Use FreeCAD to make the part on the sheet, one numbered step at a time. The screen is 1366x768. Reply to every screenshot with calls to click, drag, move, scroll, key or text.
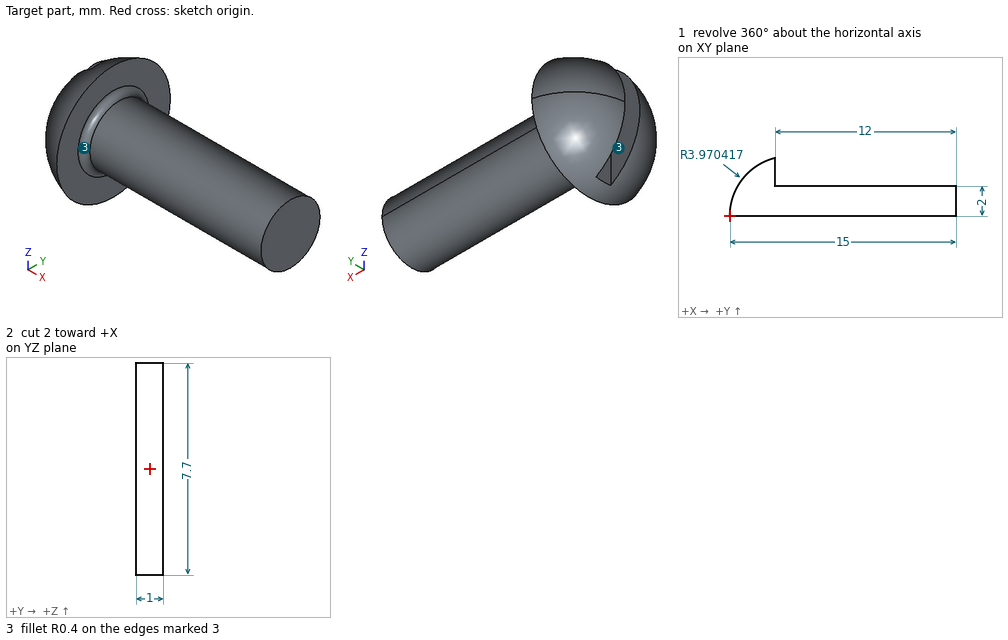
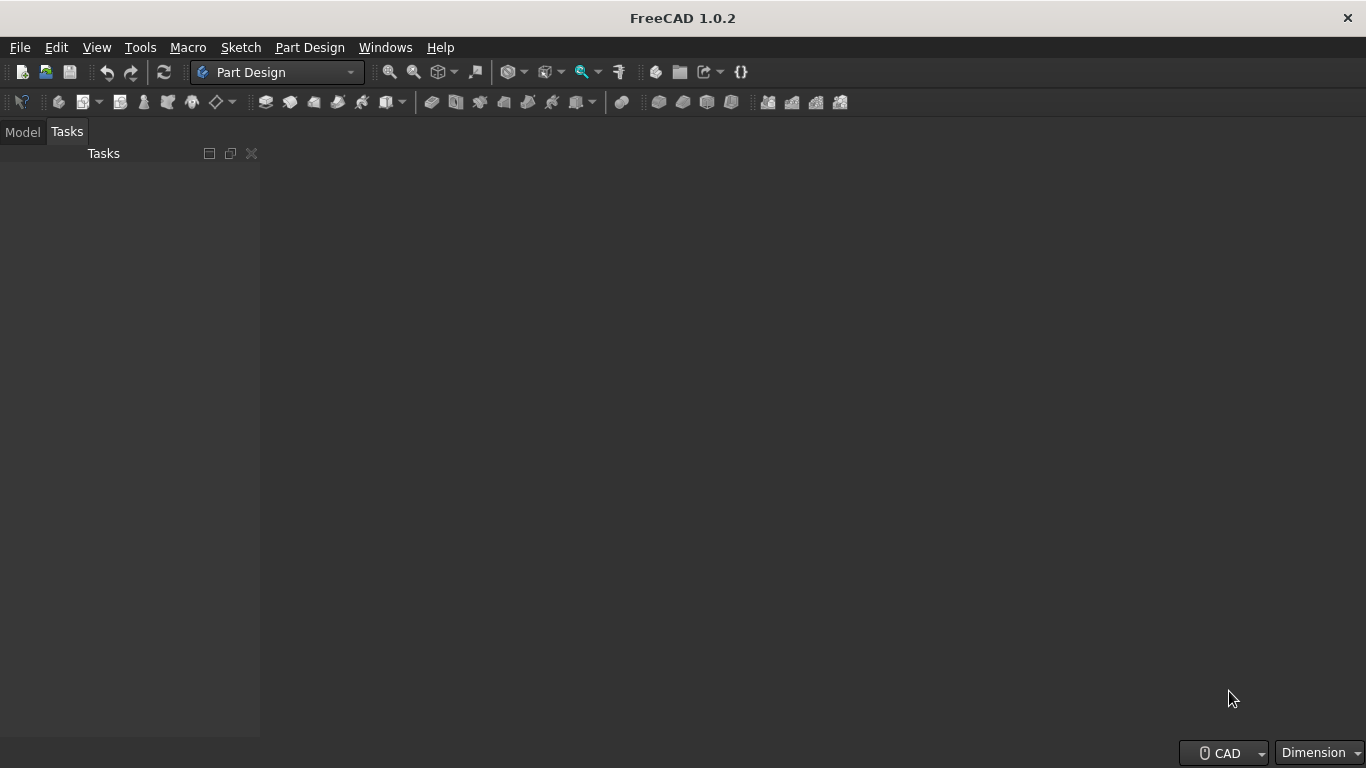
click(22, 72)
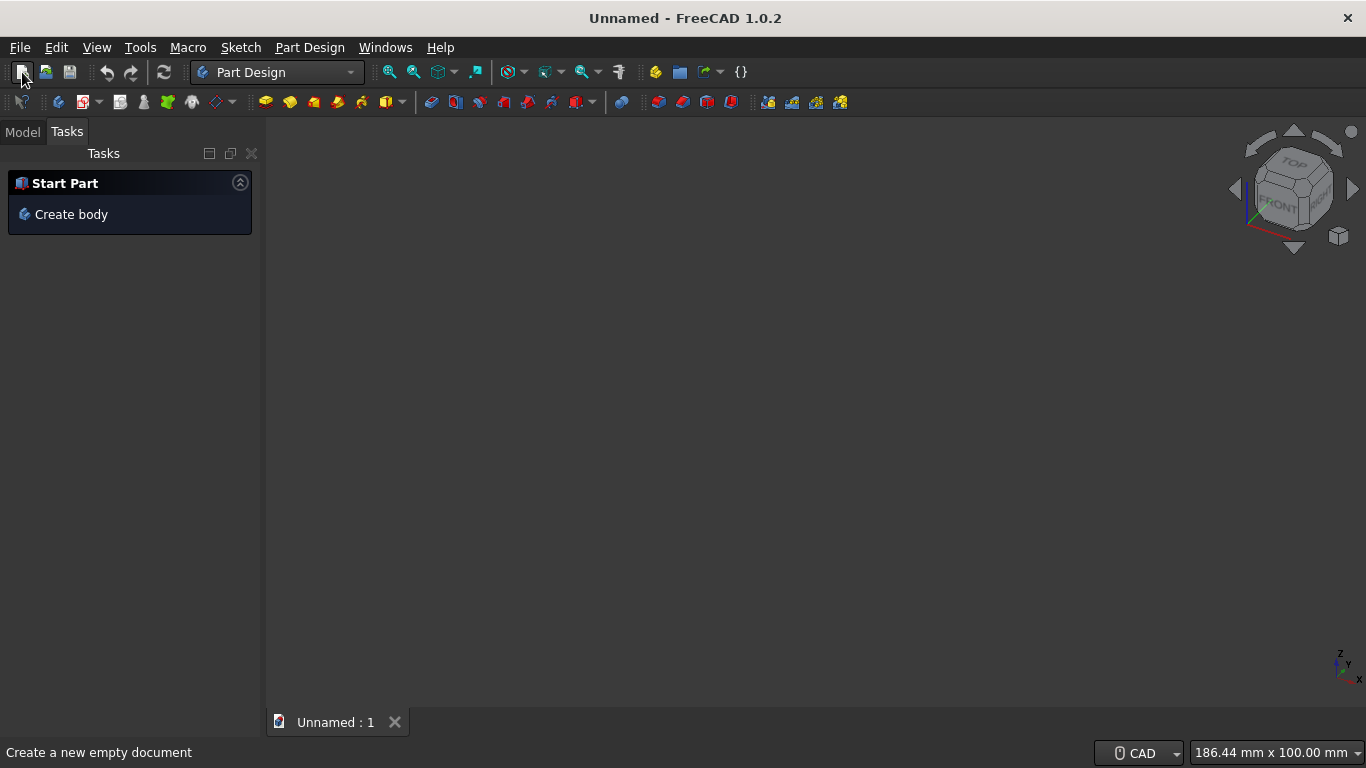
click(84, 102)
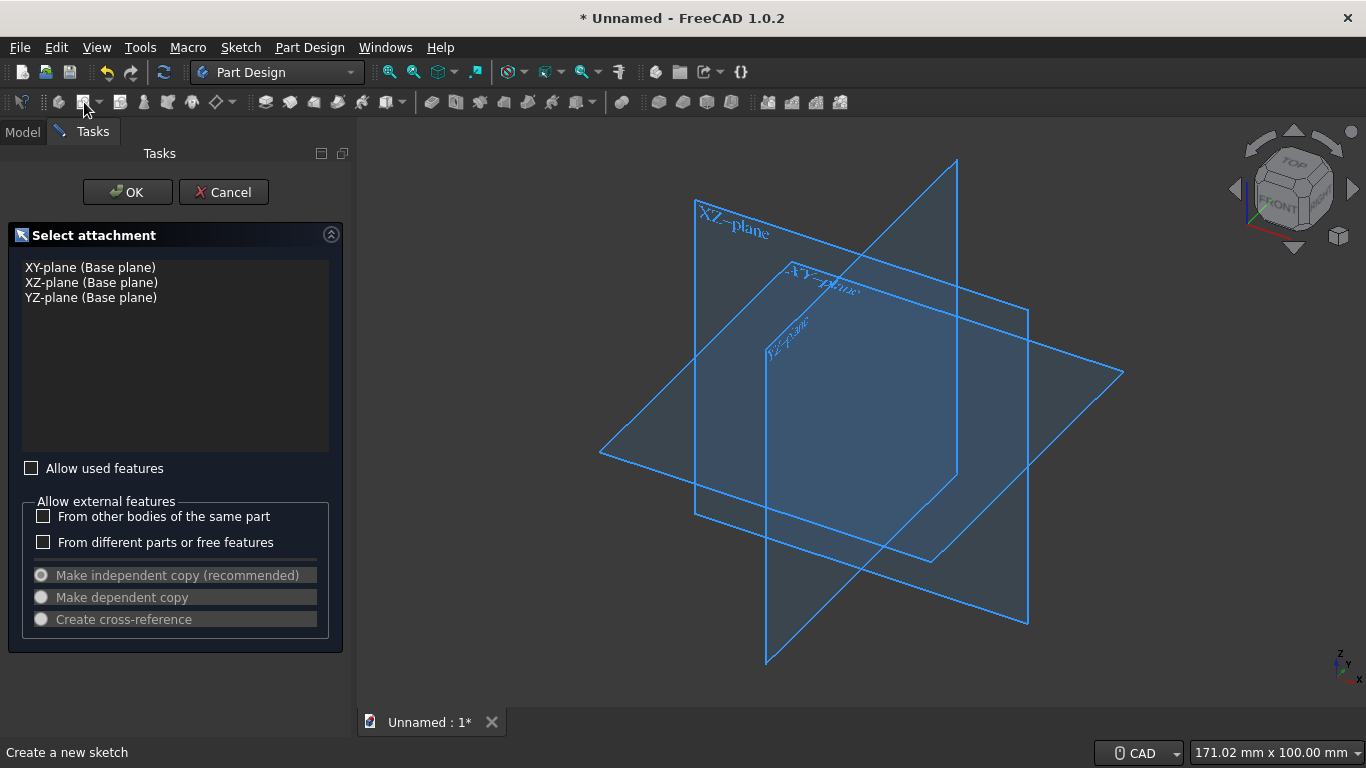
click(82, 268)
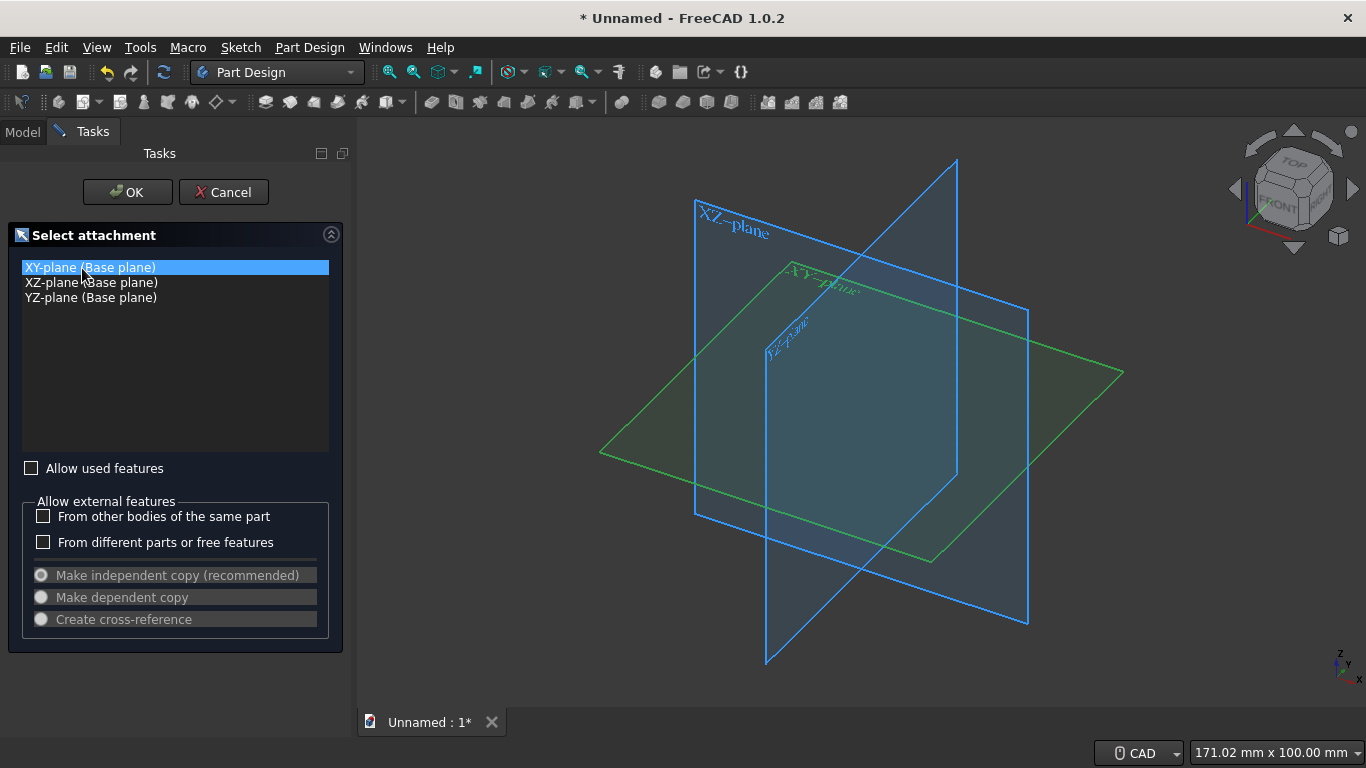
click(128, 192)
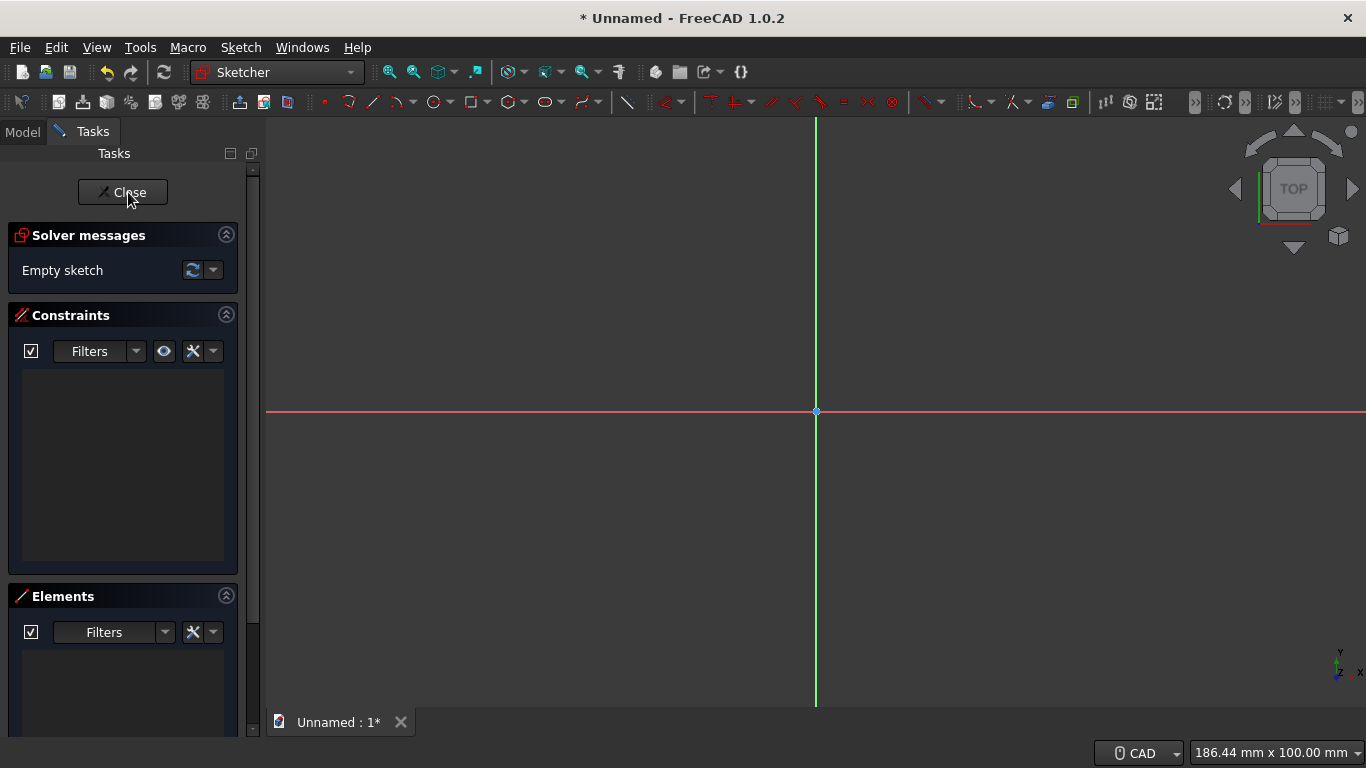
scroll(878, 399, up, 10)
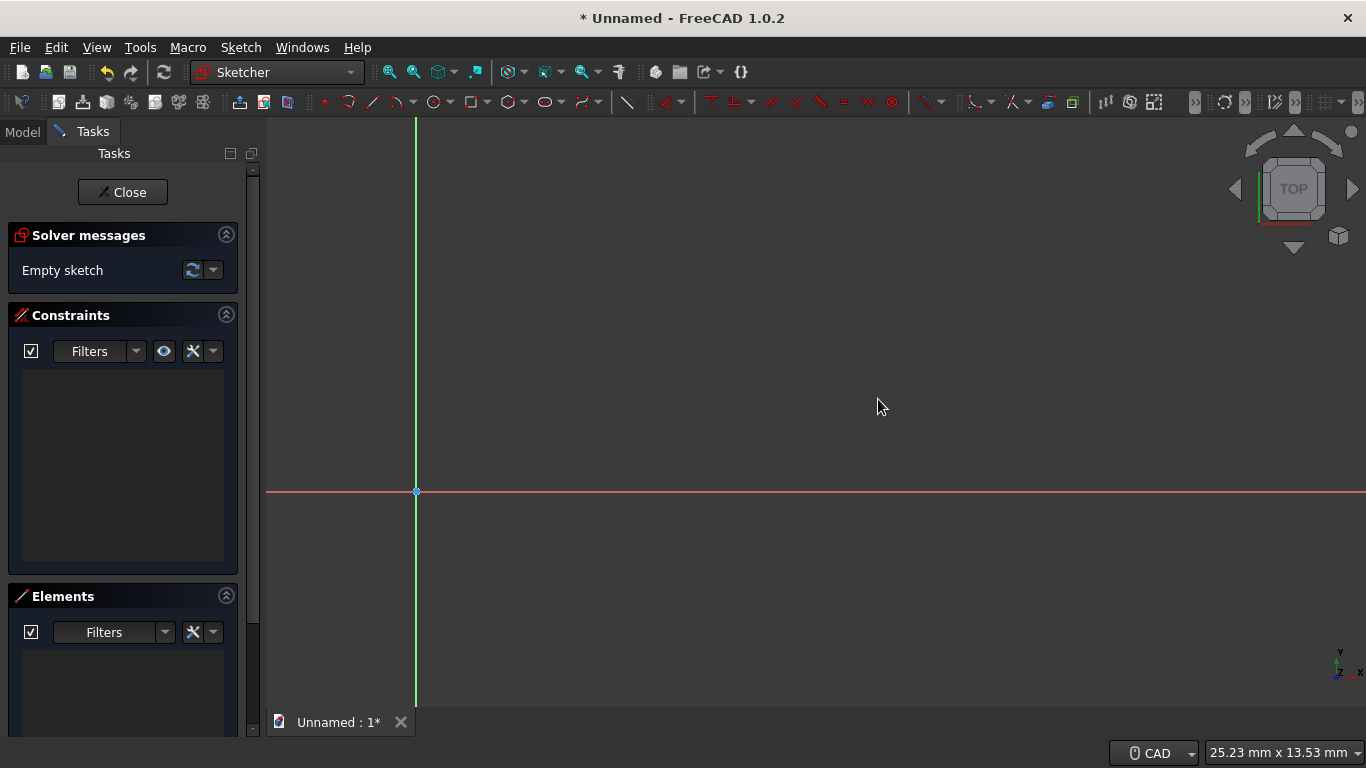
click(350, 102)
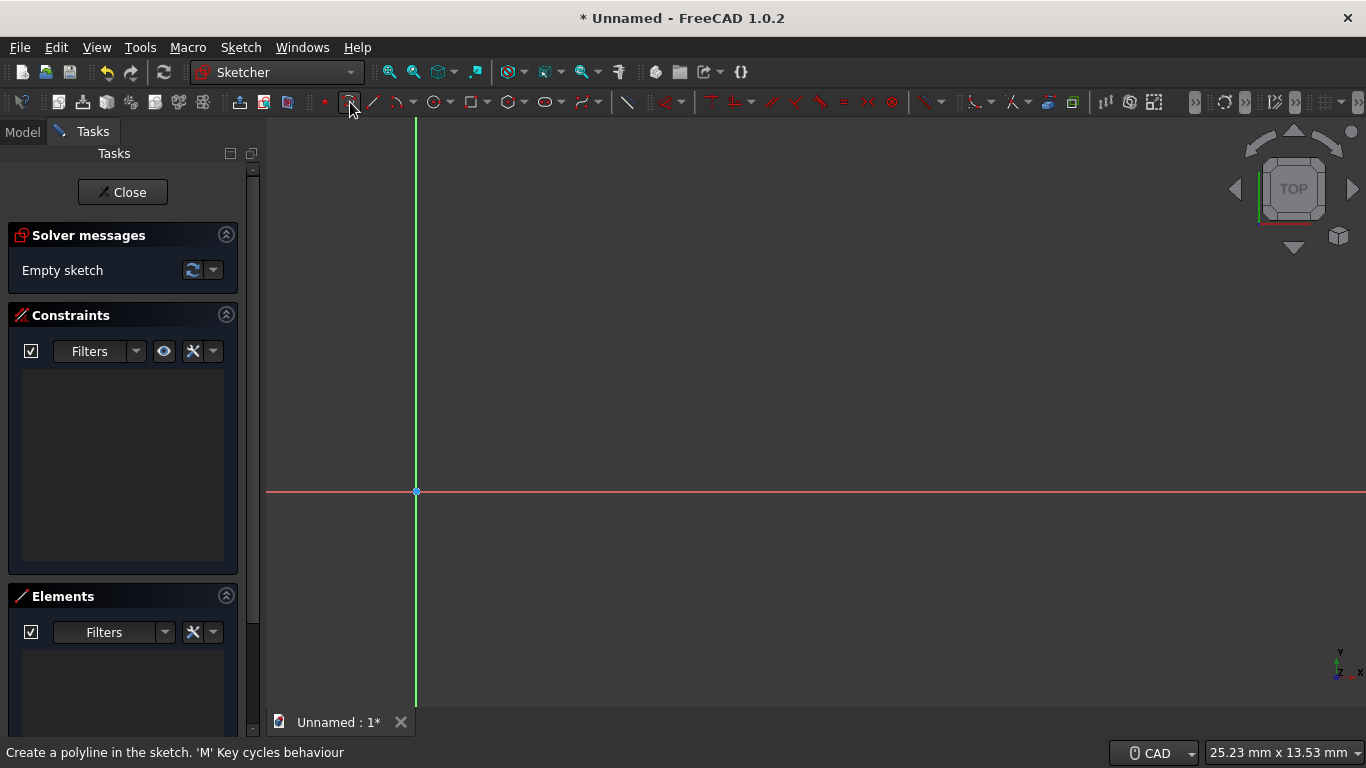
click(416, 492)
click(1070, 483)
click(1070, 405)
click(547, 405)
click(547, 324)
right_click(547, 324)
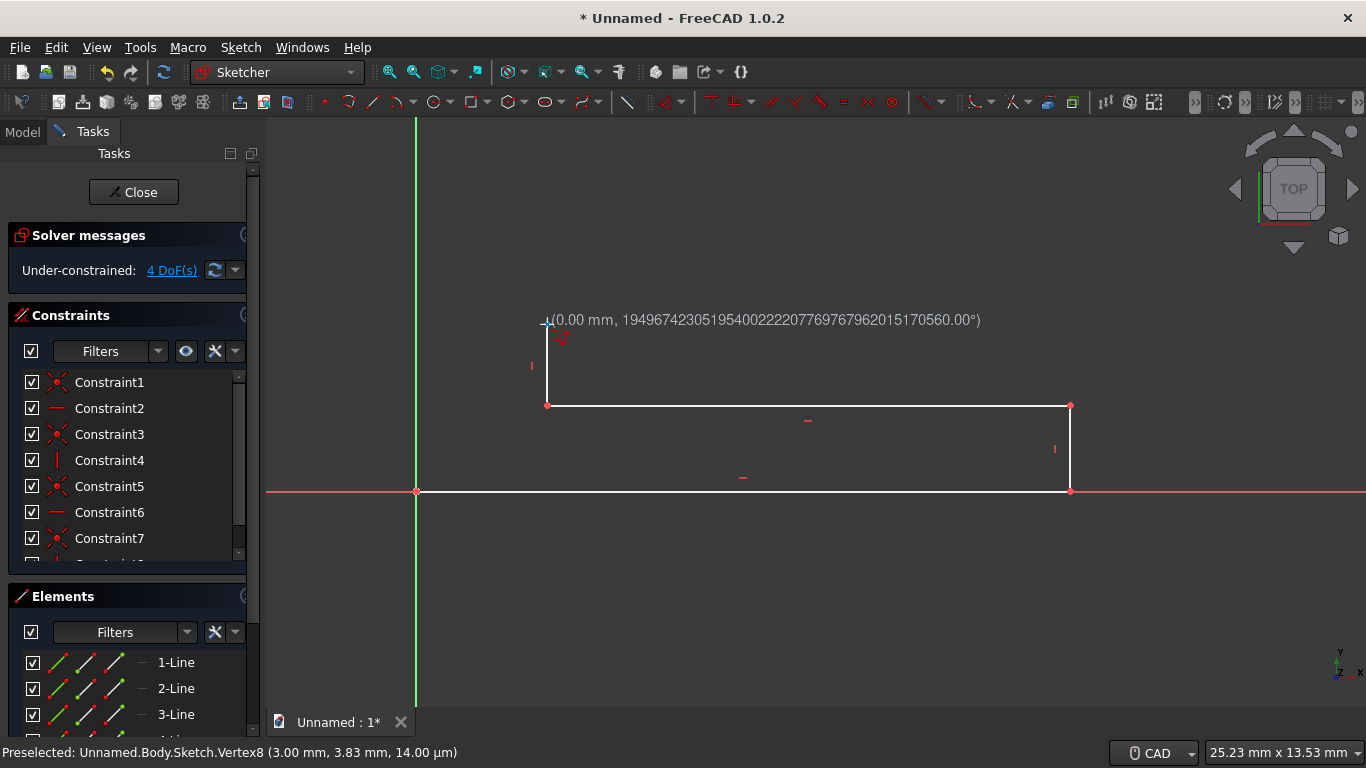
key(g)
key(3)
key(a)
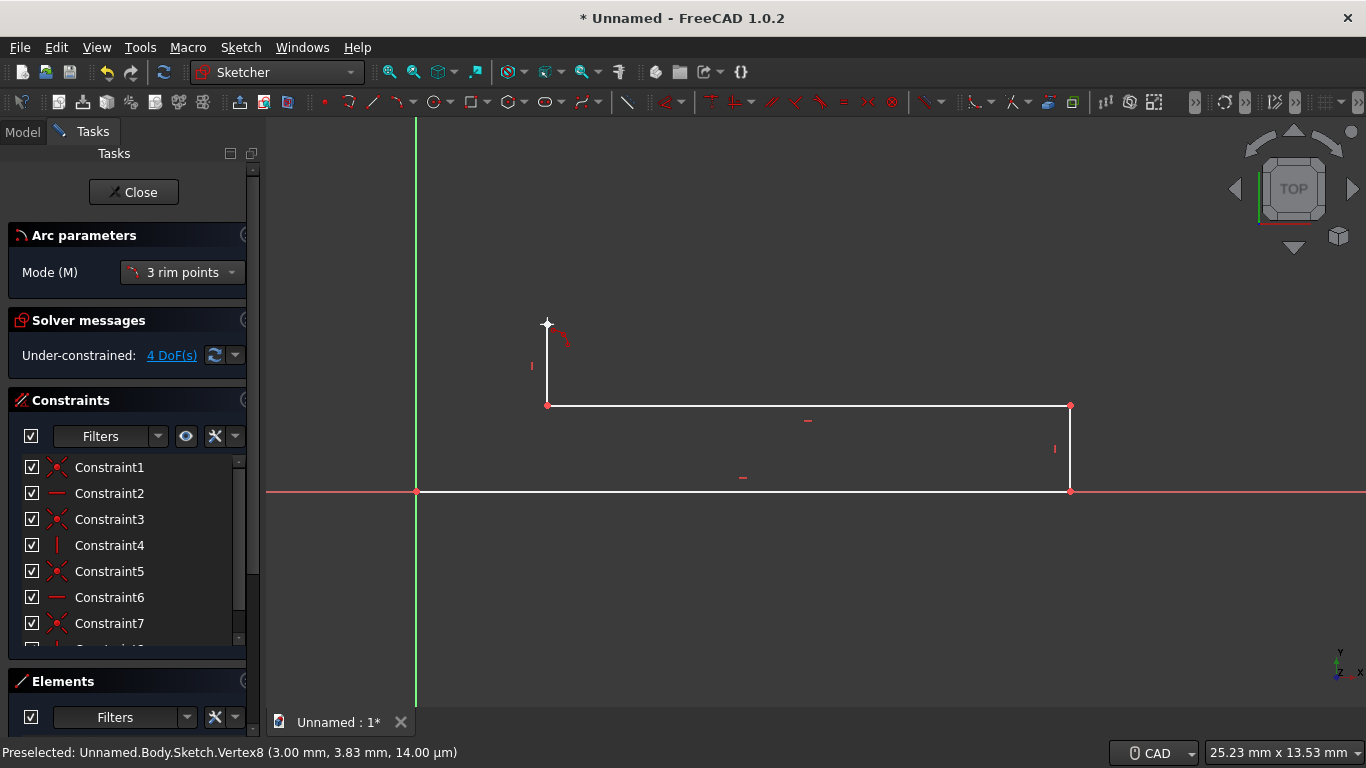
click(547, 325)
click(416, 492)
click(453, 386)
key(Escape)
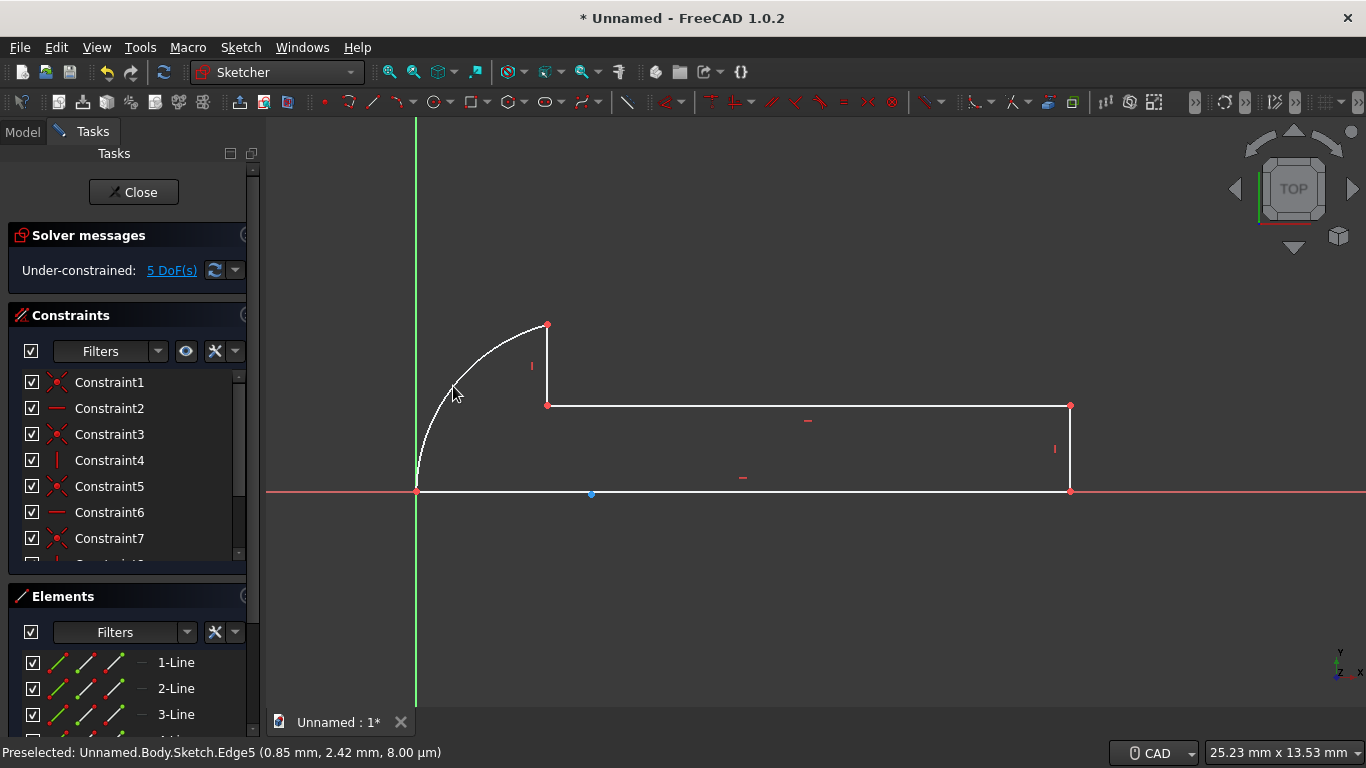
click(591, 494)